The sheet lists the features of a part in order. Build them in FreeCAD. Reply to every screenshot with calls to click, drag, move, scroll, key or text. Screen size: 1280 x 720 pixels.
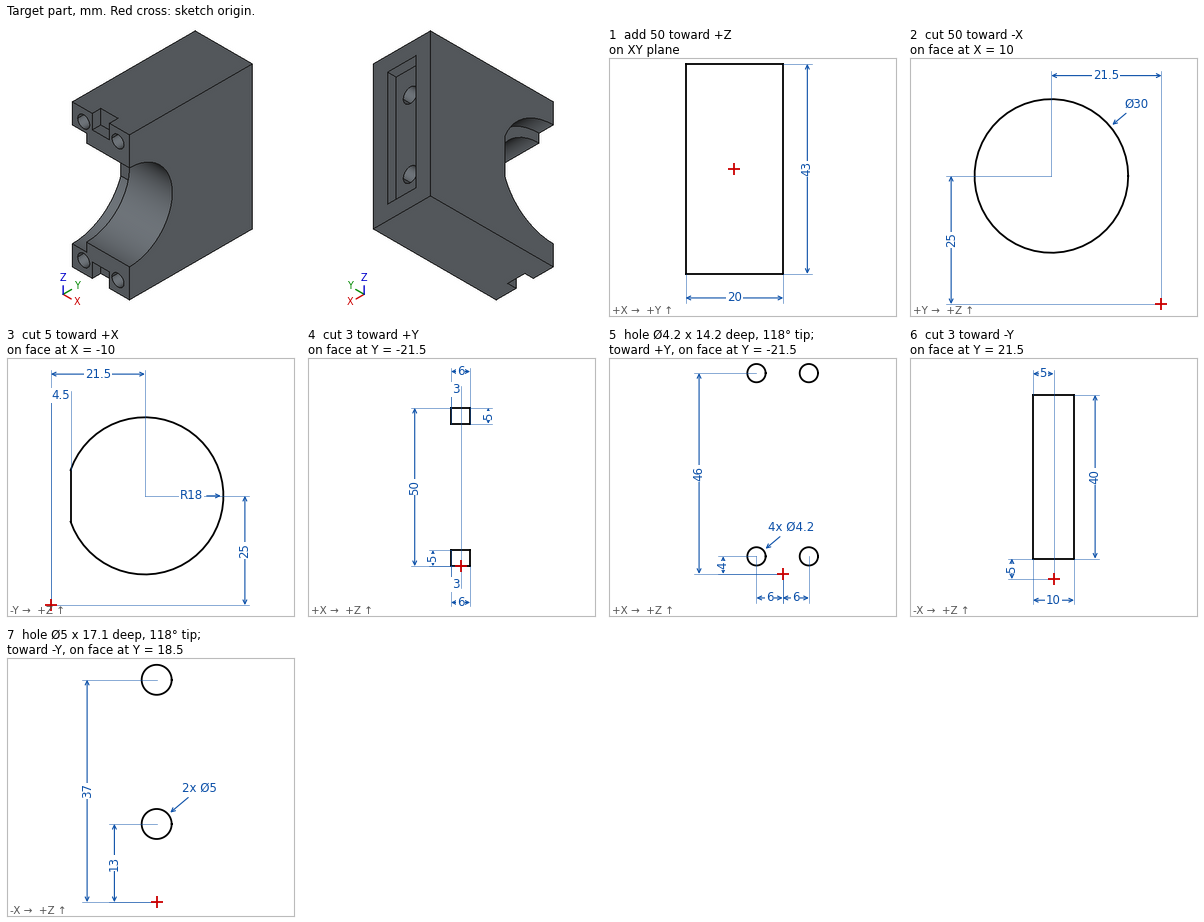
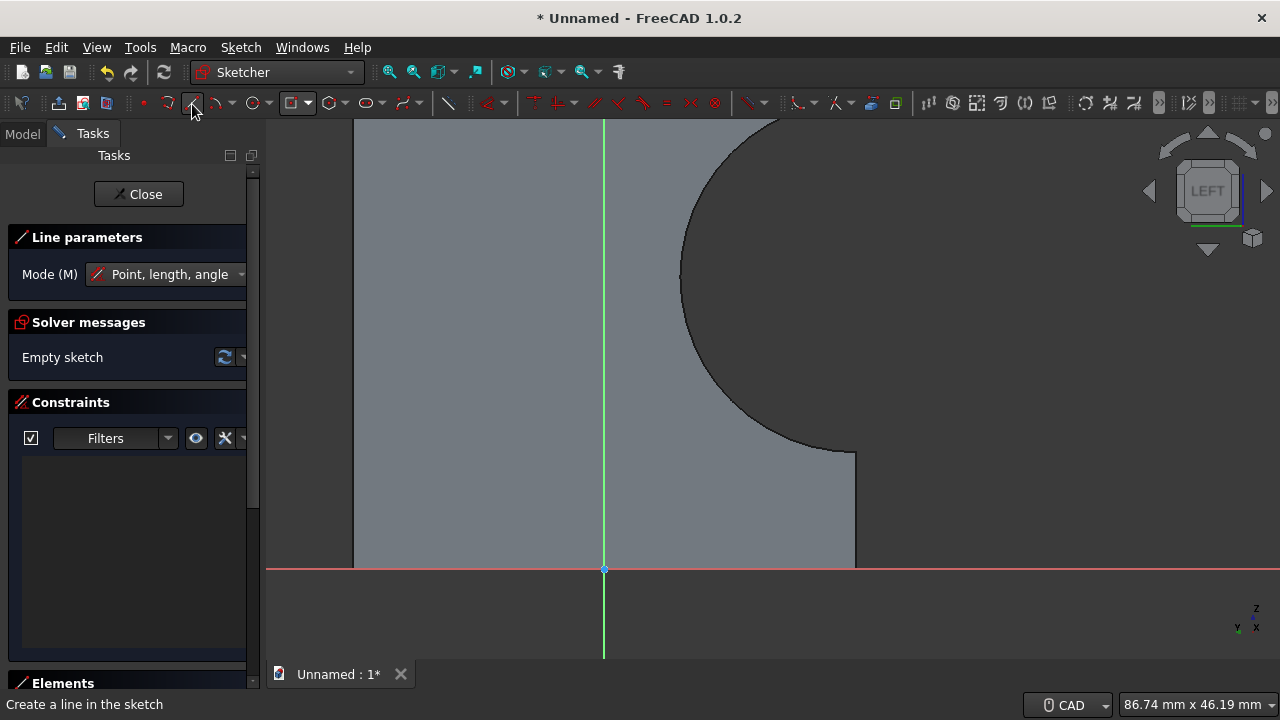
click(657, 208)
click(657, 346)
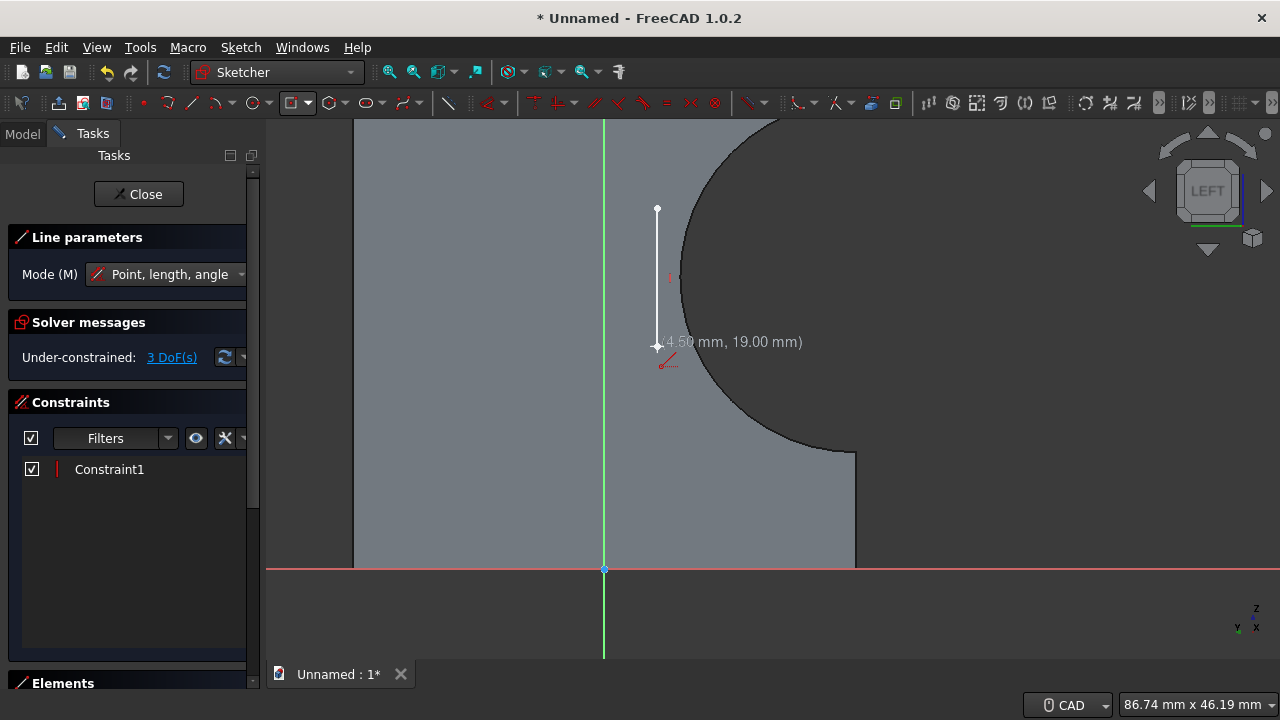
key(g)
key(3)
key(a)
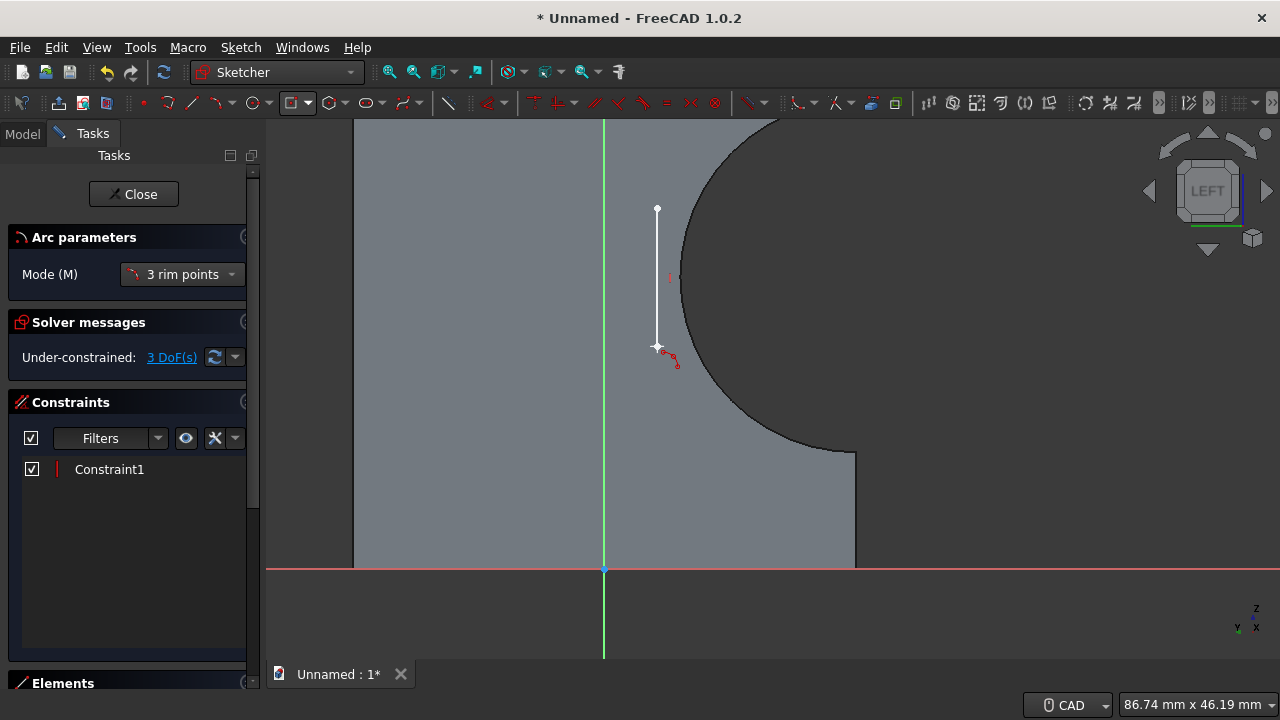
click(657, 347)
click(657, 209)
click(1066, 277)
key(Escape)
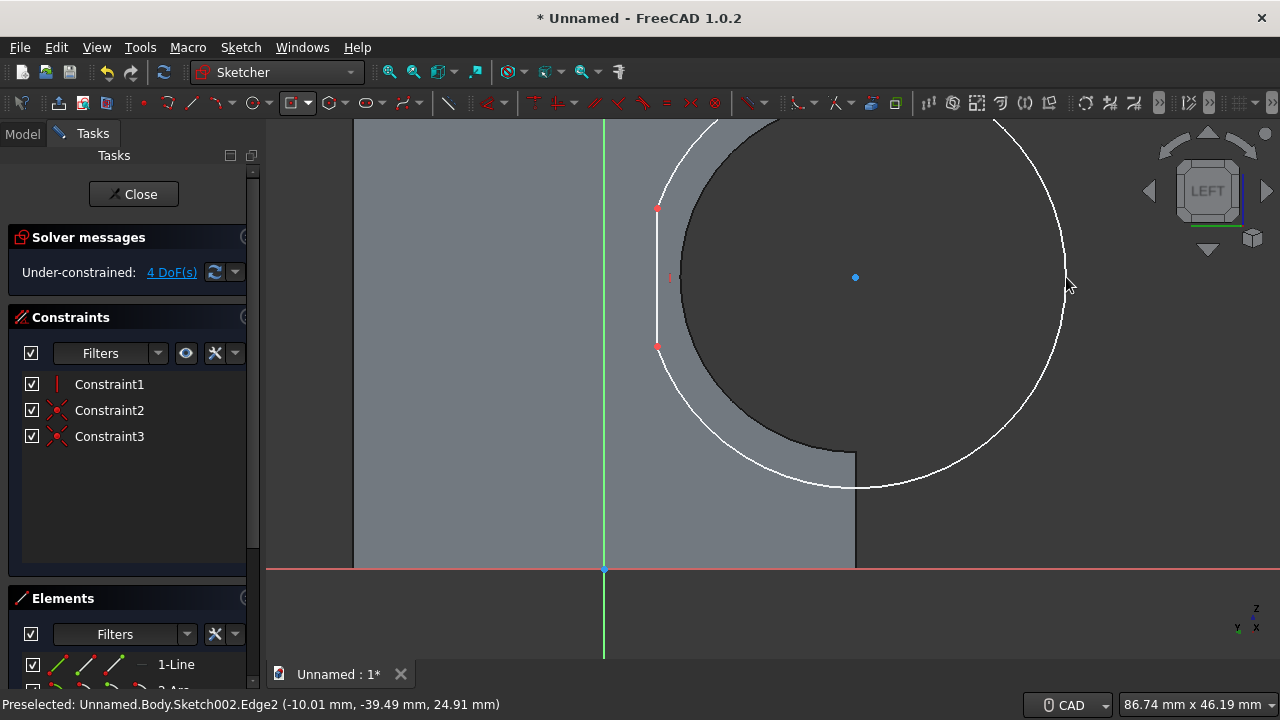
click(488, 104)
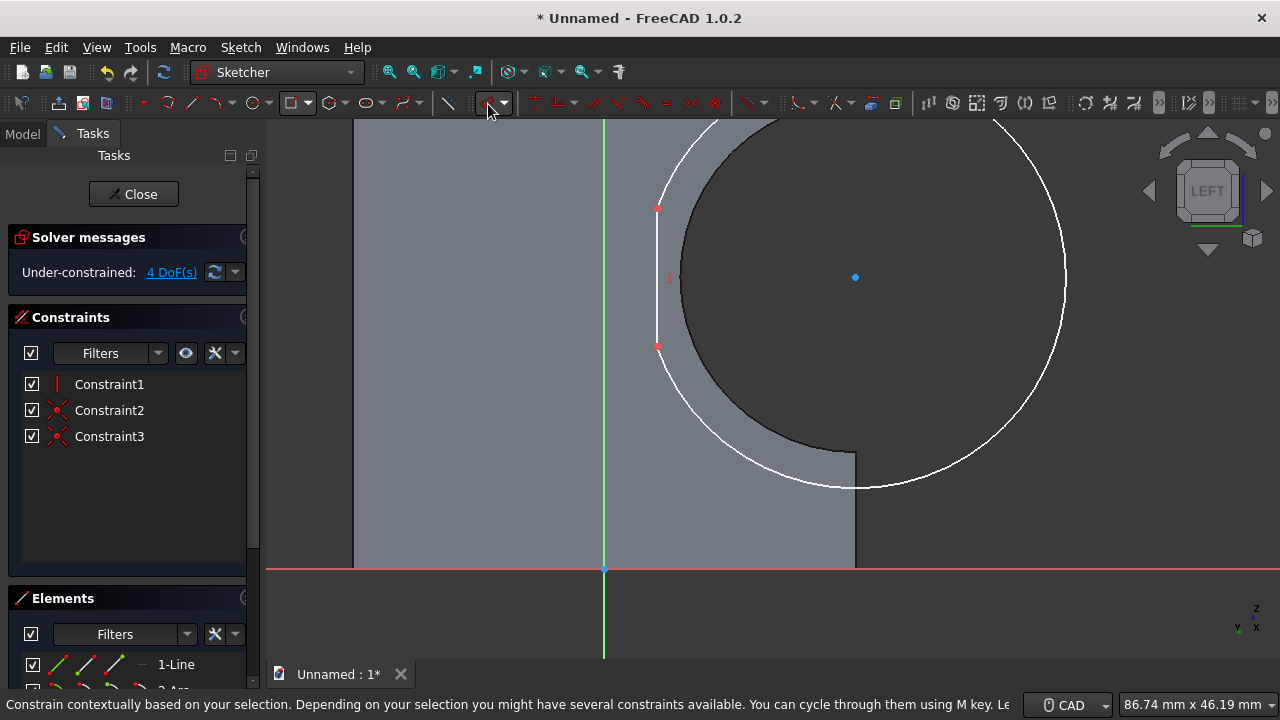
click(947, 468)
click(961, 497)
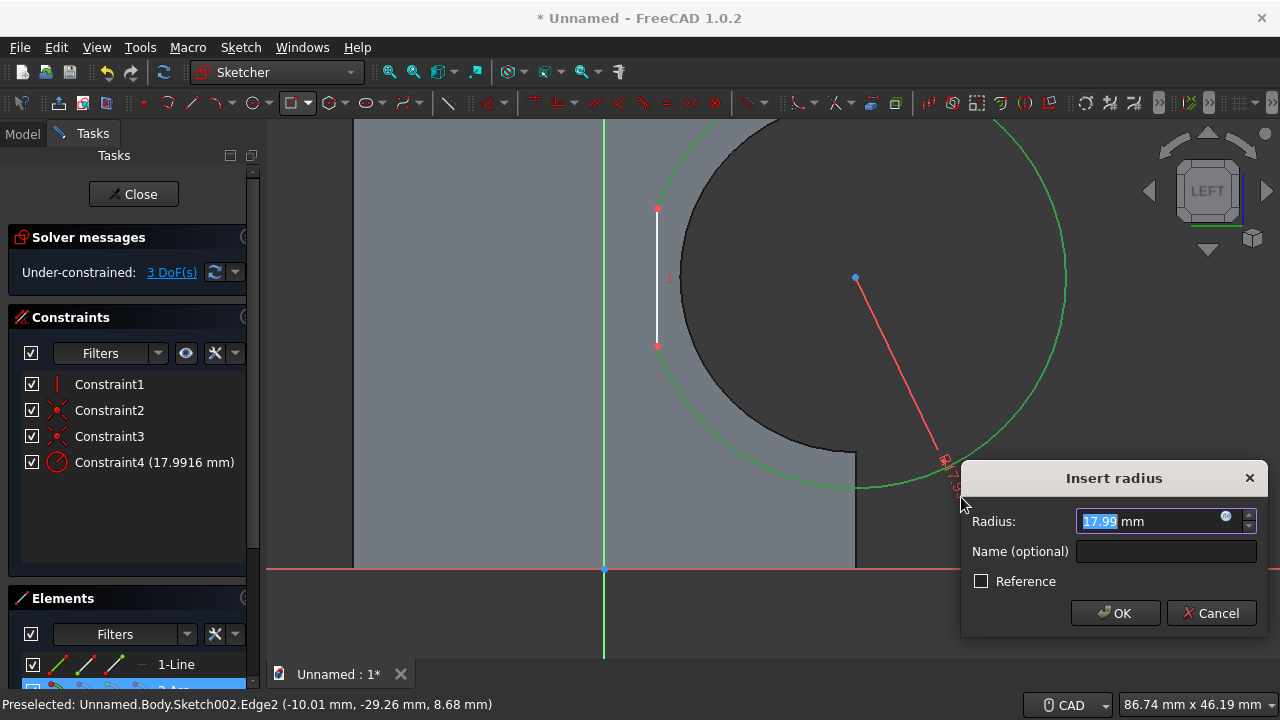
text(18)
key(Return)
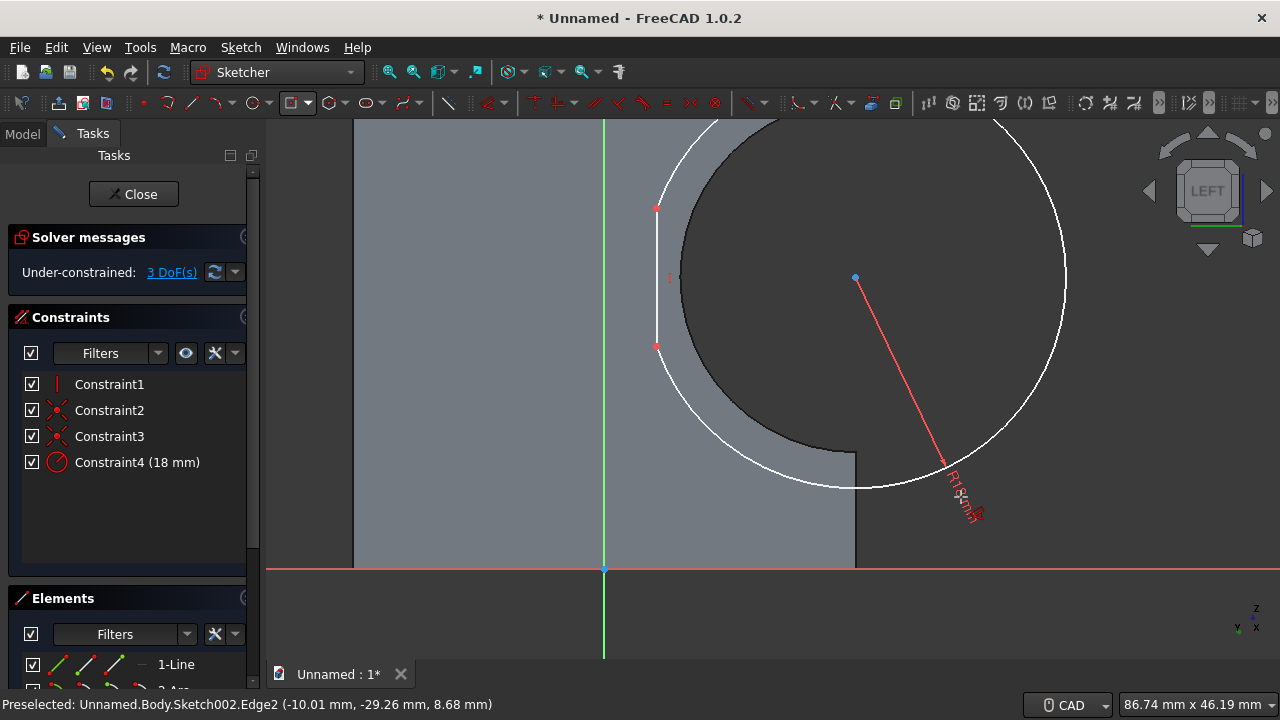
click(856, 278)
click(570, 424)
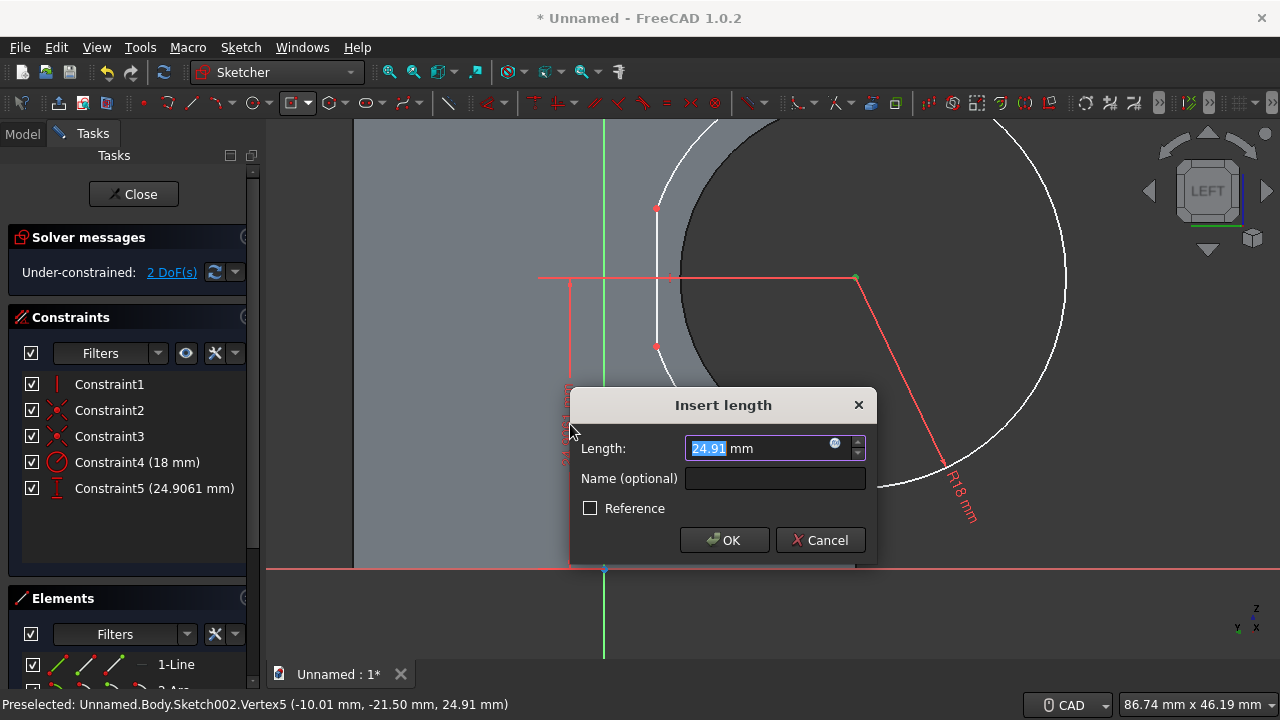
text(25)
key(Return)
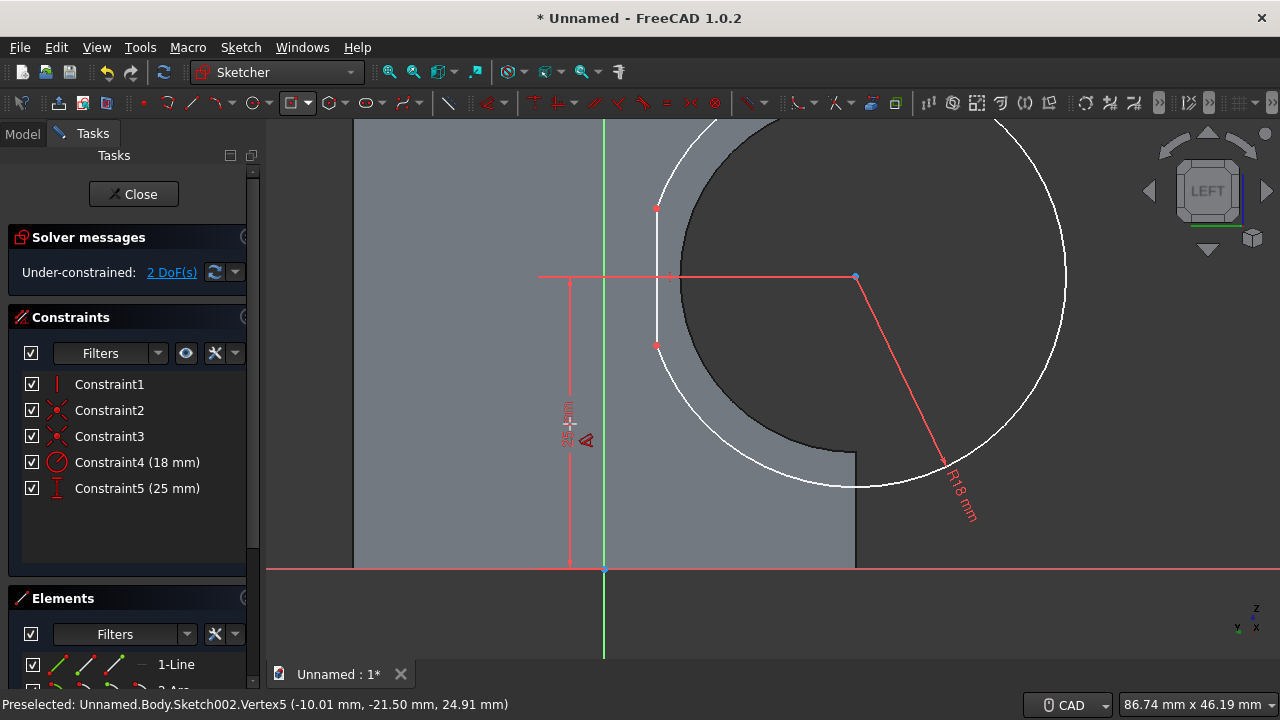
click(657, 208)
click(631, 603)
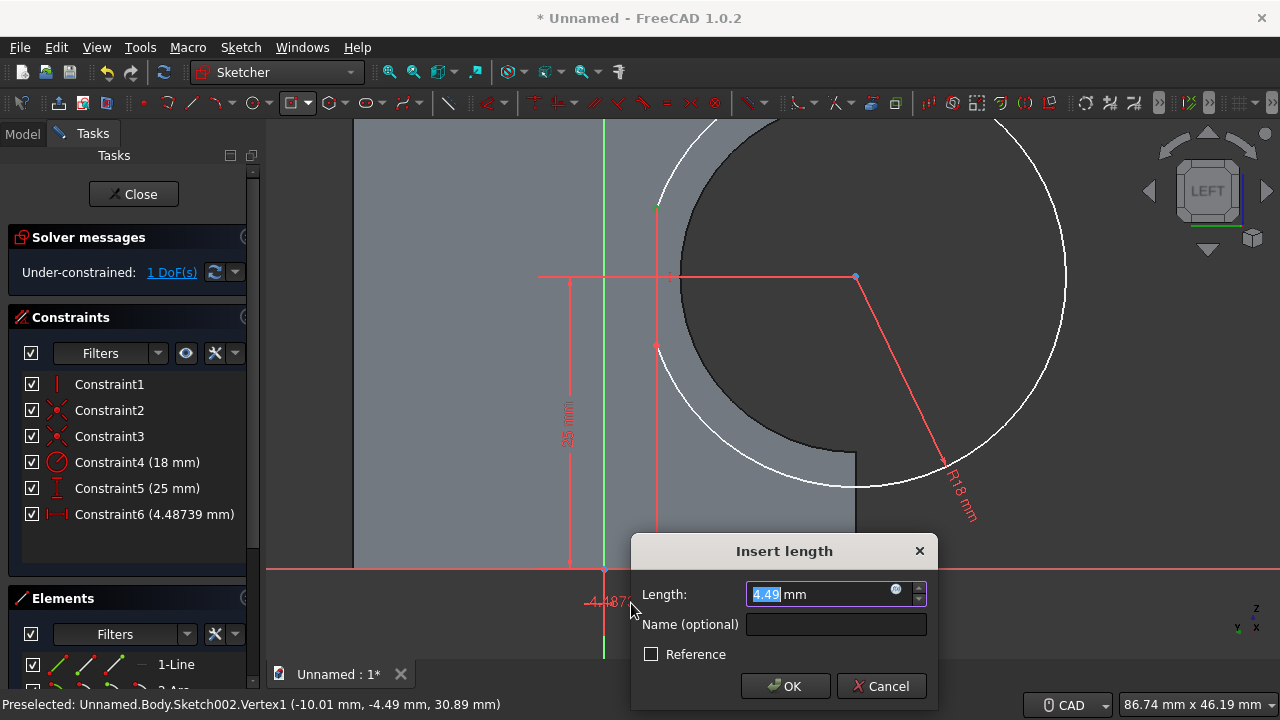
text(4.5)
key(Return)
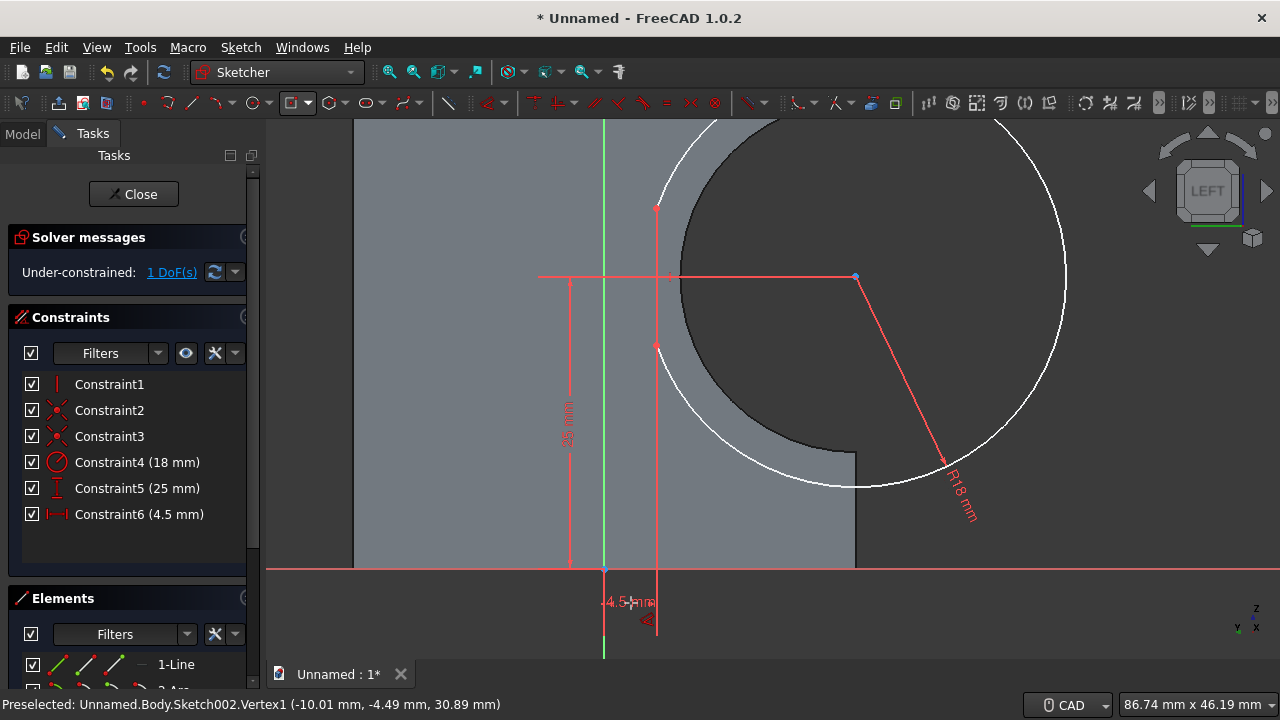
click(856, 277)
click(730, 603)